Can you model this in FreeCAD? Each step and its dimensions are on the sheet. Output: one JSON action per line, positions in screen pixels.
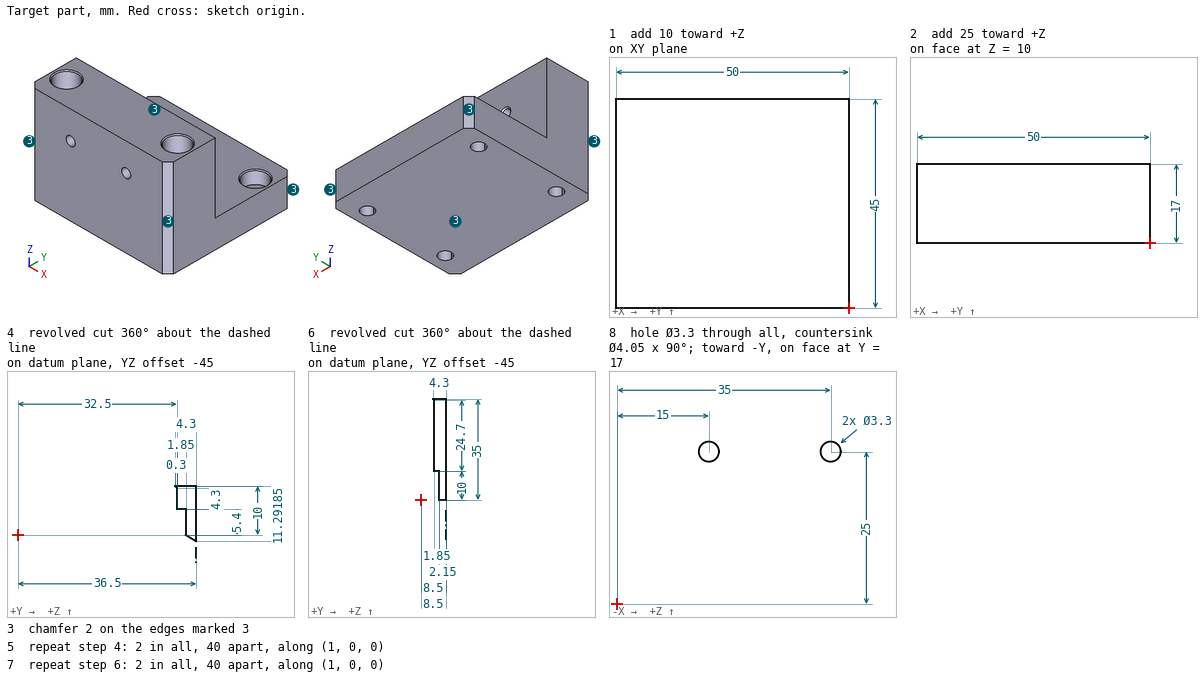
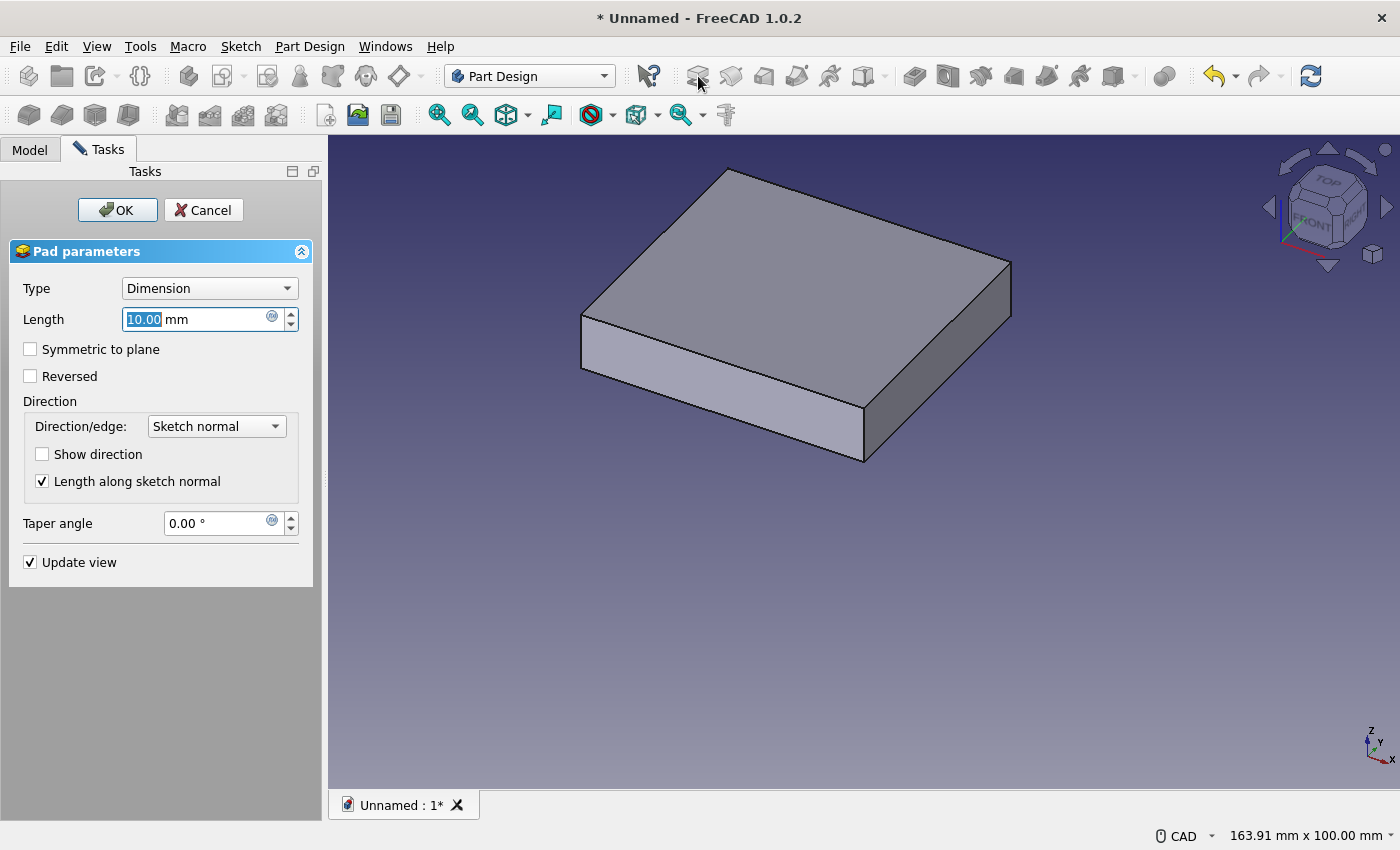
{"action": "type", "text": "10"}
{"action": "key", "text": "Tab"}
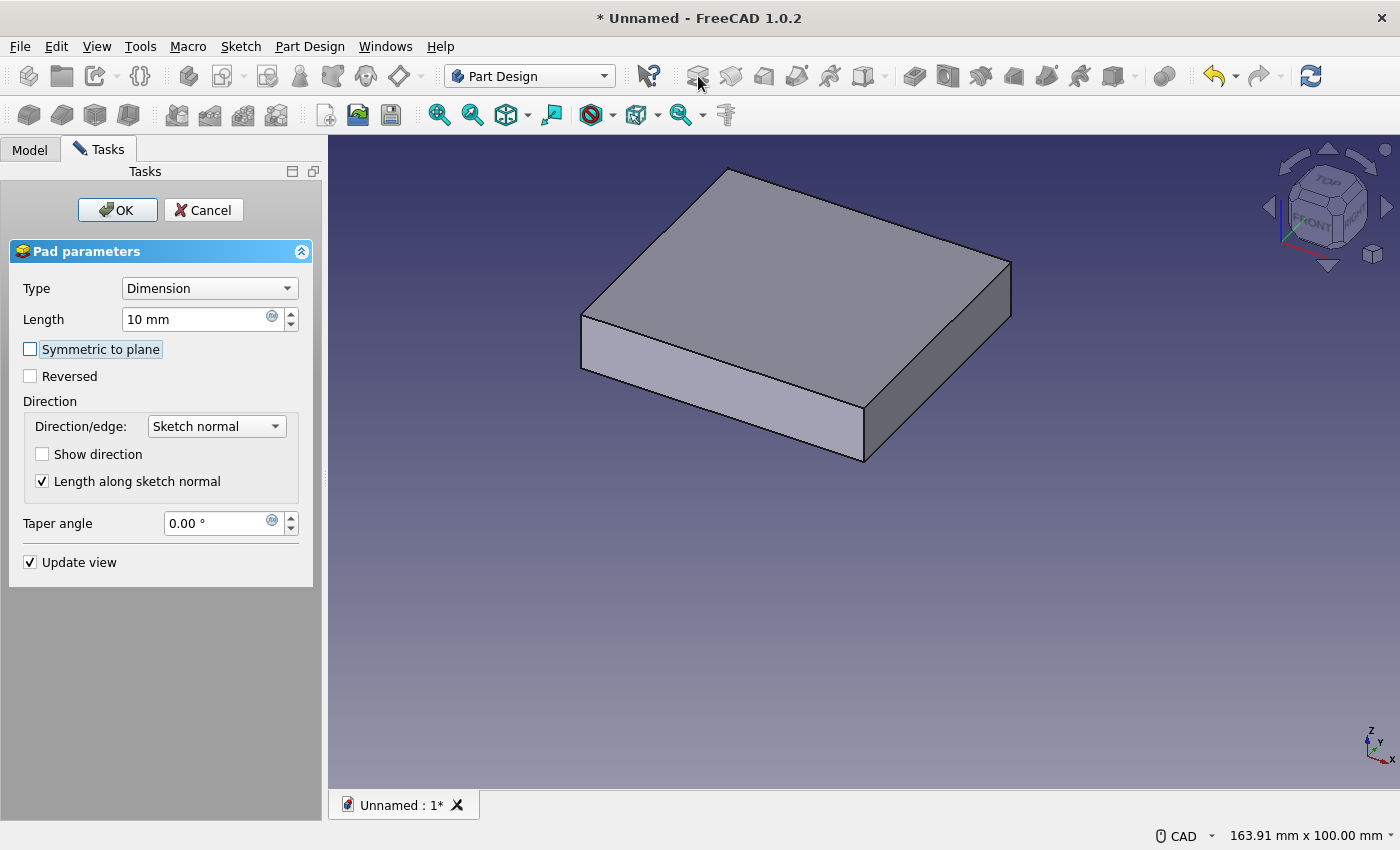
{"action": "left_click", "coordinate": [118, 210]}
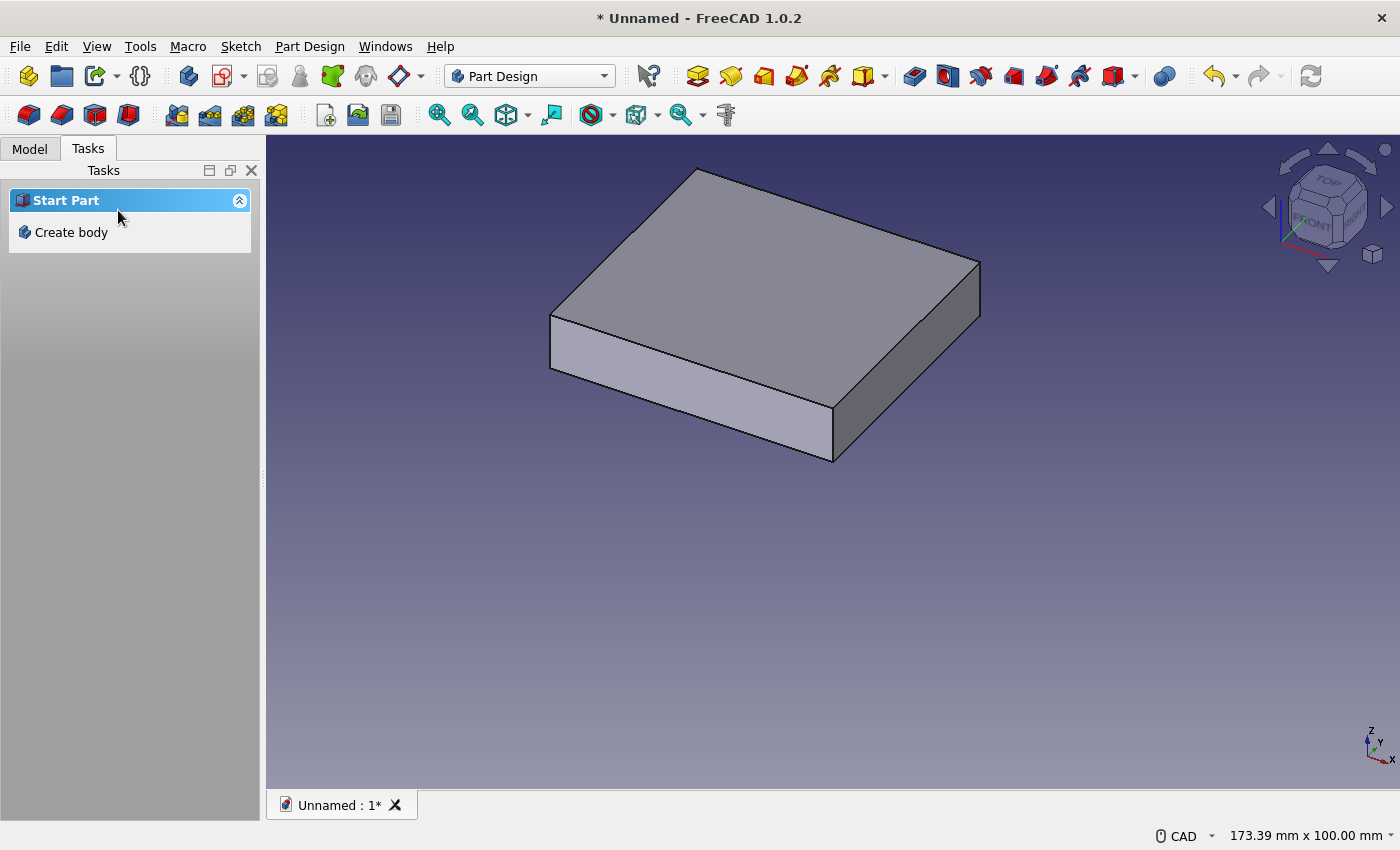
{"action": "key", "text": "v f"}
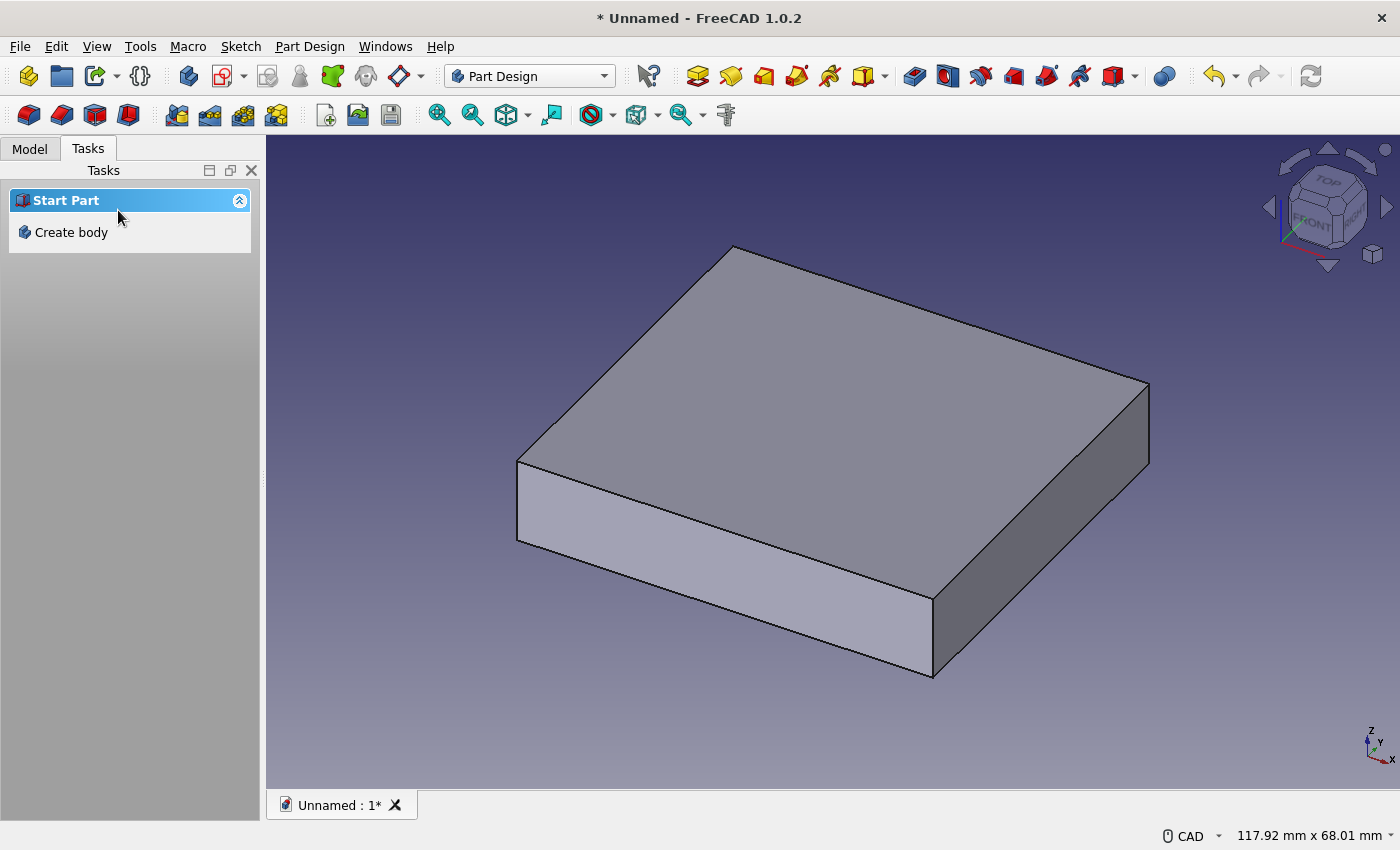
{"action": "left_click", "coordinate": [833, 422]}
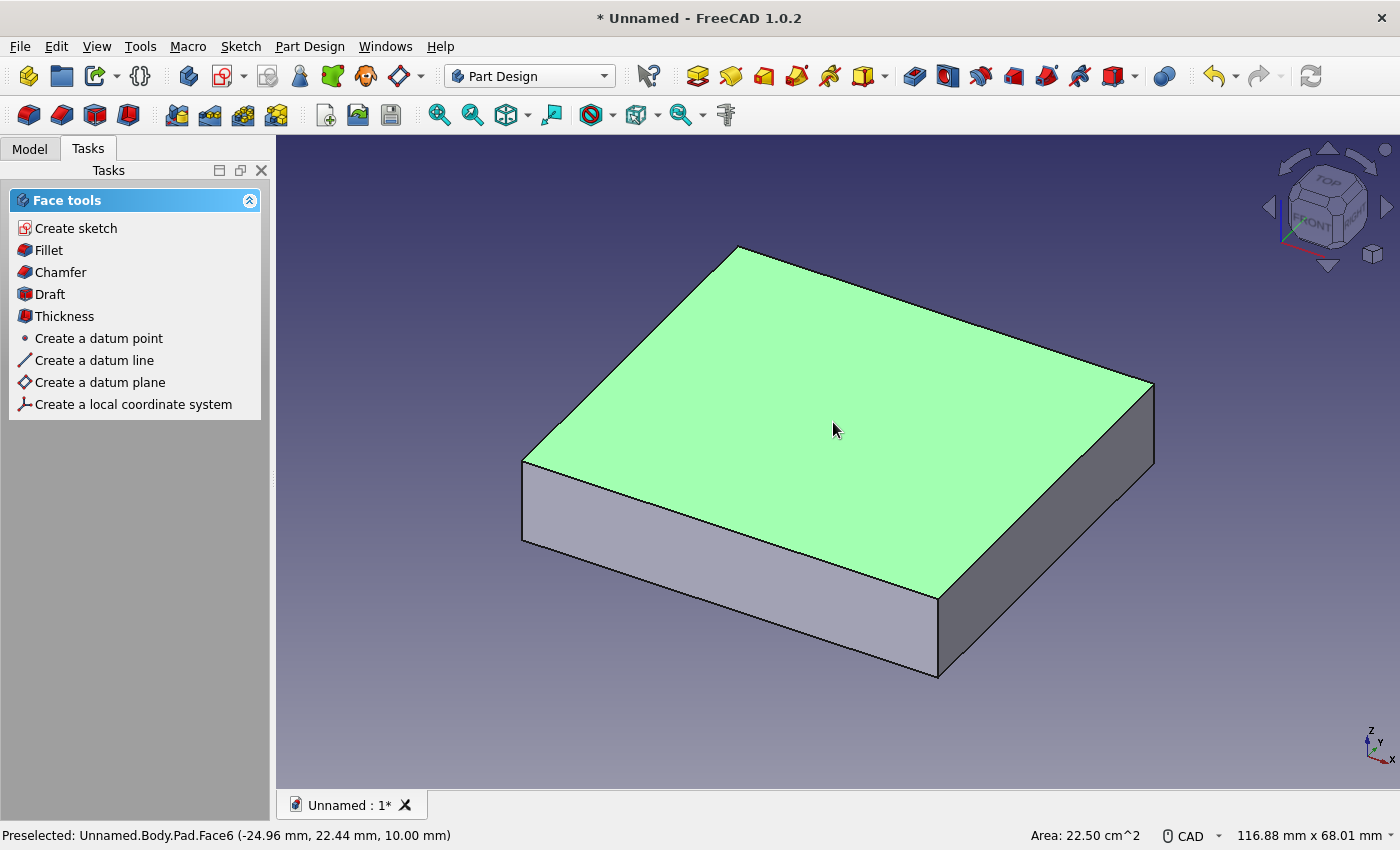
{"action": "left_click", "coordinate": [222, 76]}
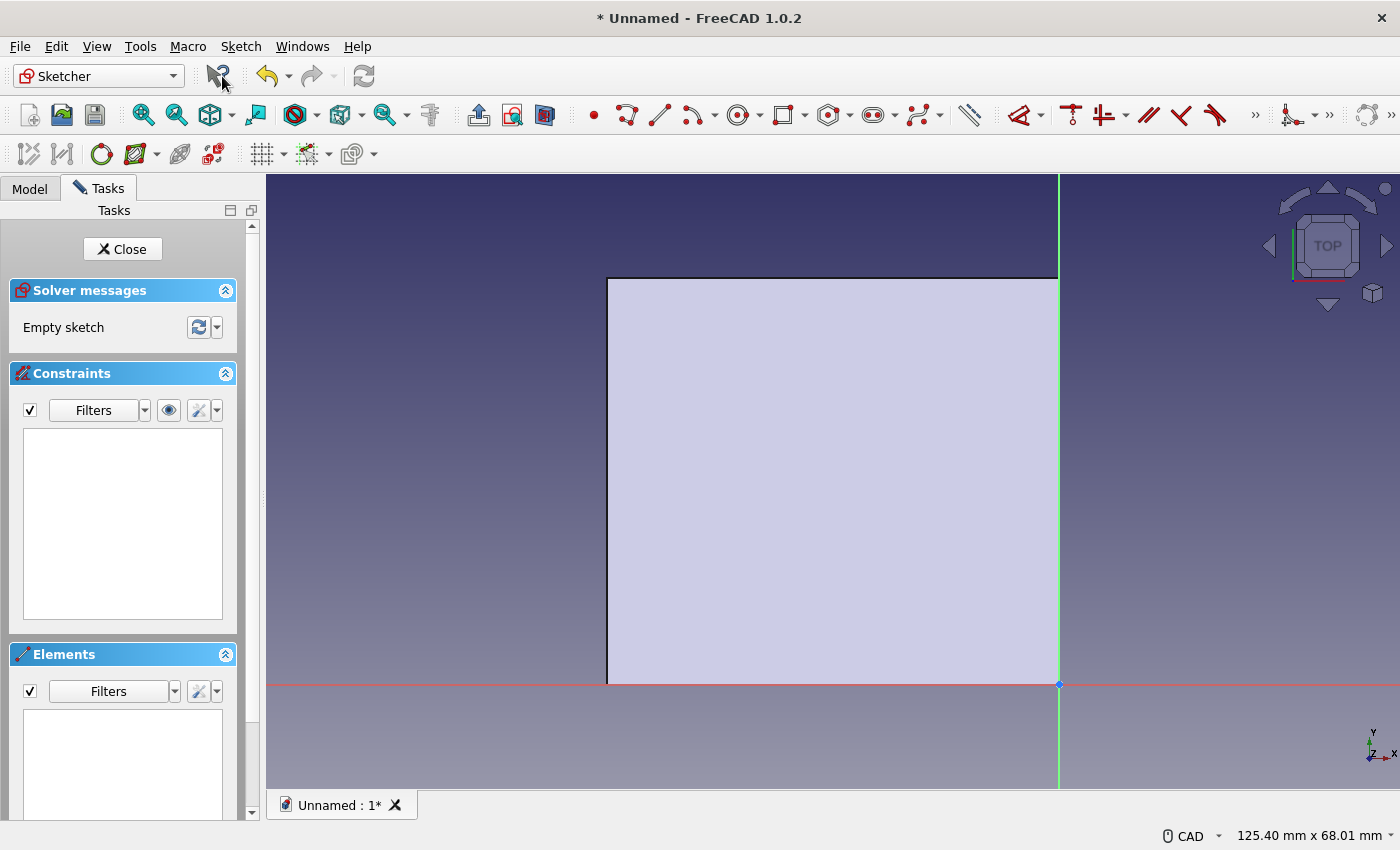
{"action": "scroll", "coordinate": [972, 761], "scroll_direction": "up", "scroll_amount": 2}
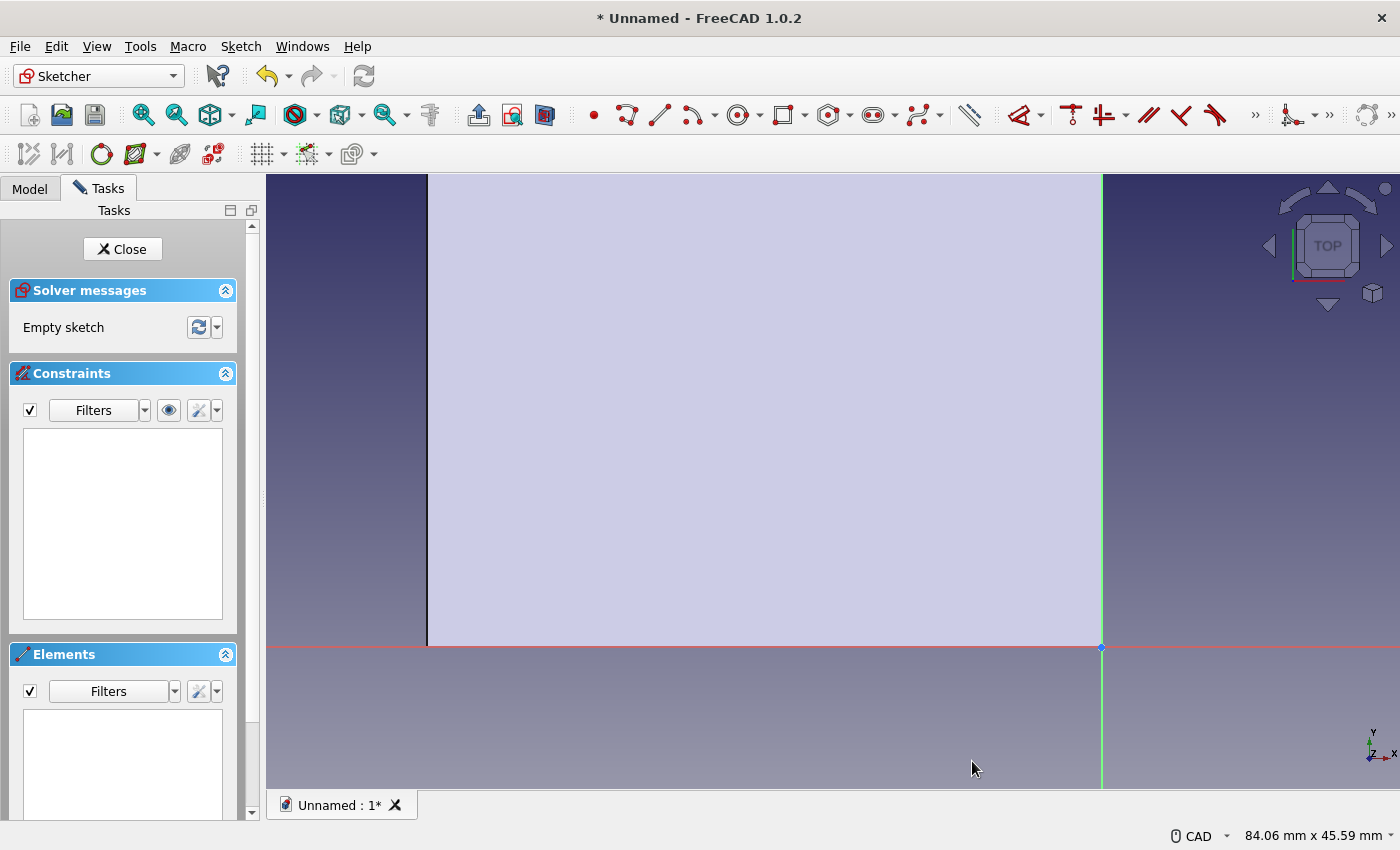
{"action": "key", "text": "g r"}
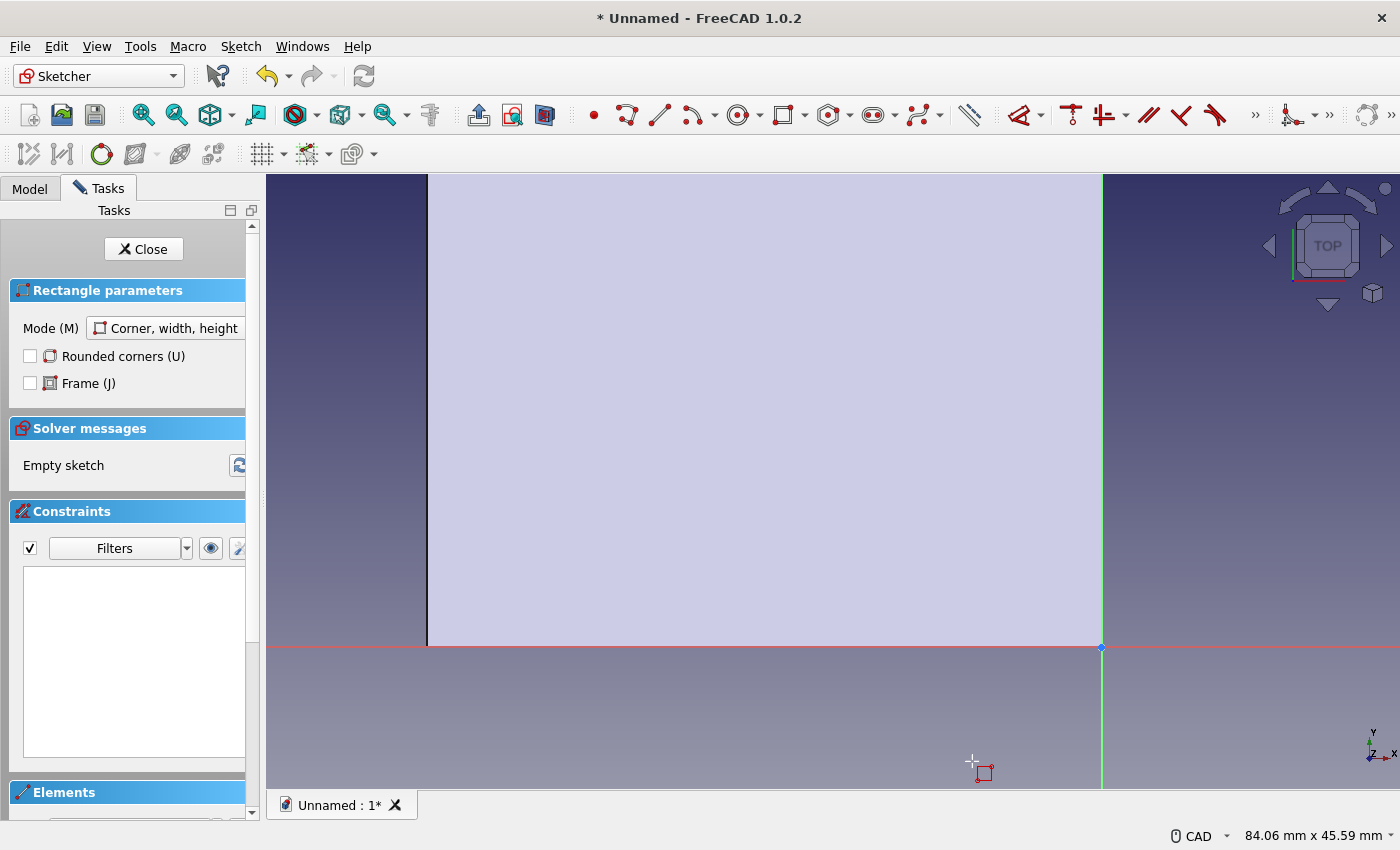
{"action": "left_click", "coordinate": [1102, 647]}
{"action": "left_click", "coordinate": [427, 418]}
{"action": "key", "text": "Escape"}